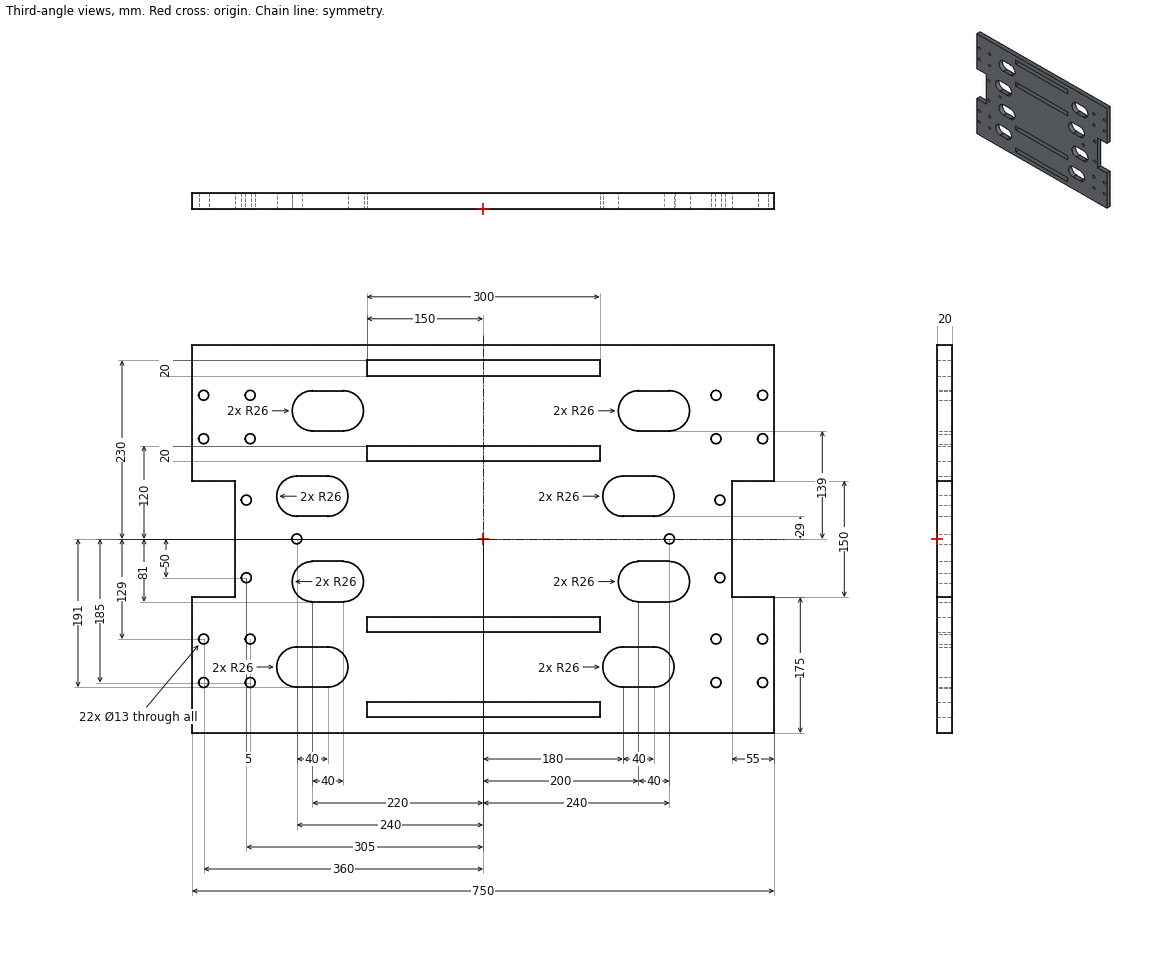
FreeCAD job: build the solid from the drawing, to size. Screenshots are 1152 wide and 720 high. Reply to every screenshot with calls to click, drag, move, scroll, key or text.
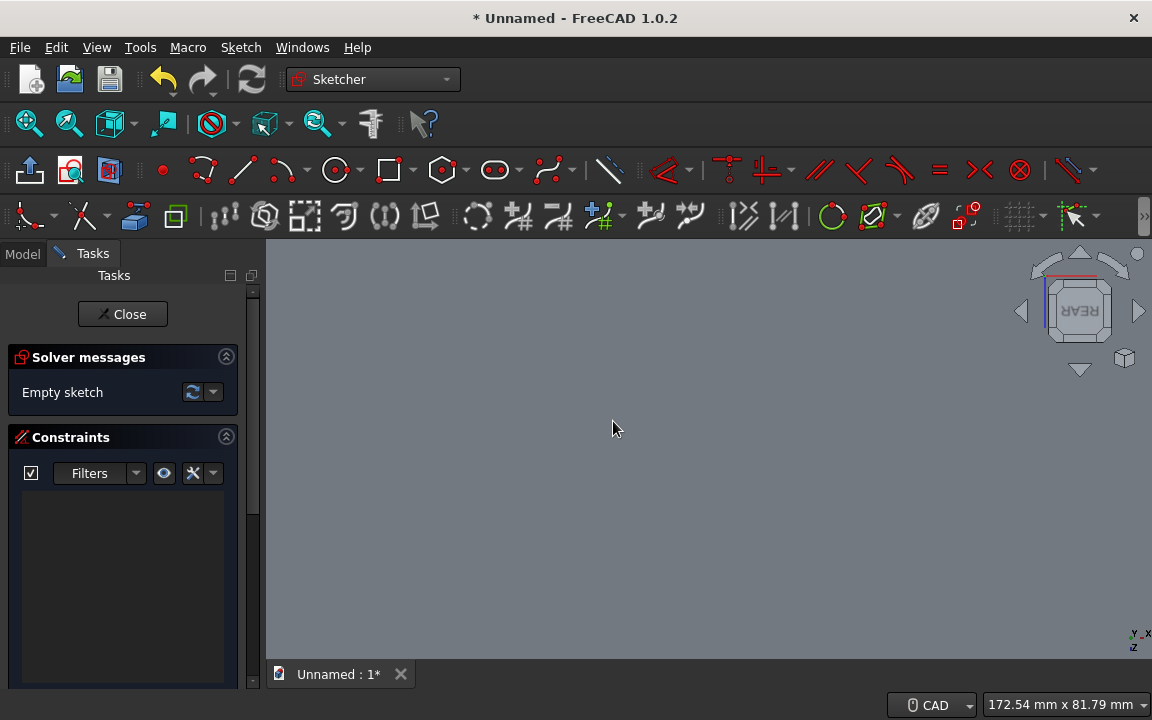
click(496, 170)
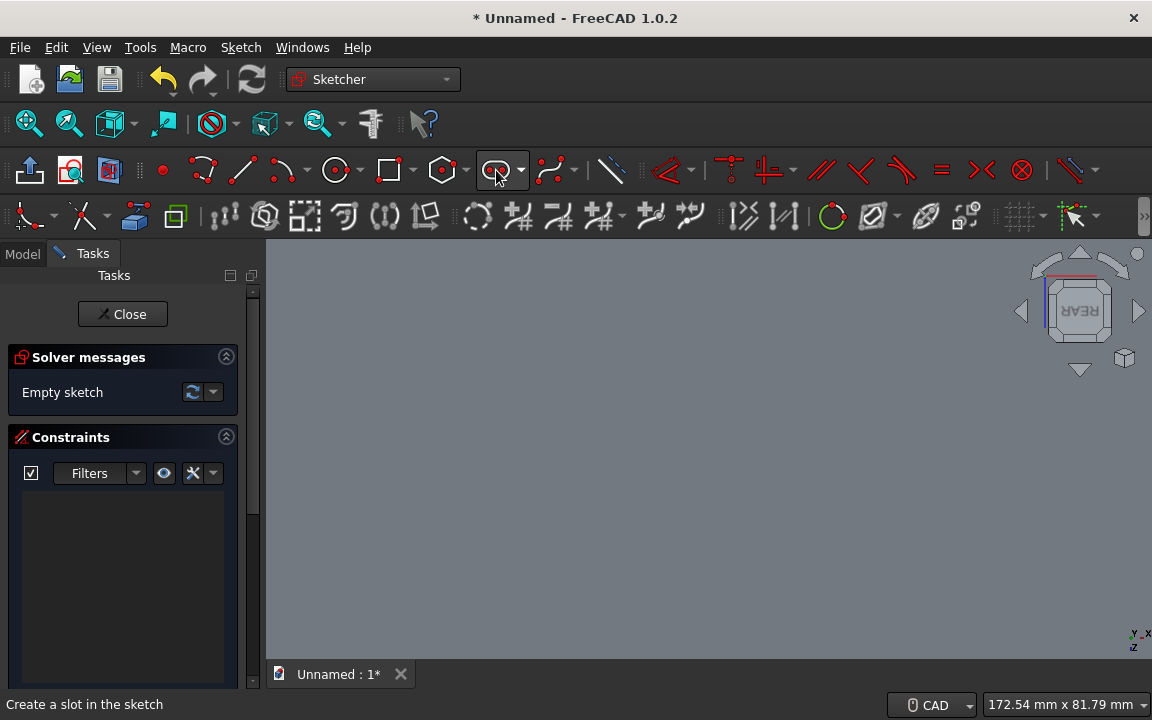
click(538, 443)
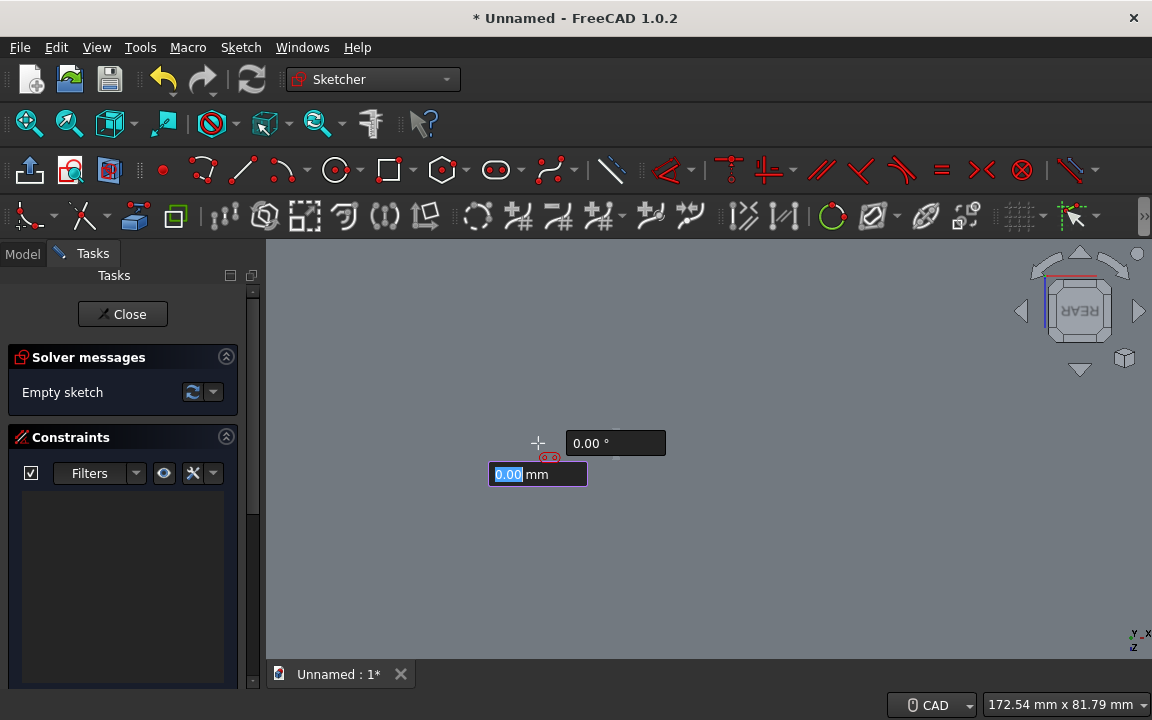
click(743, 443)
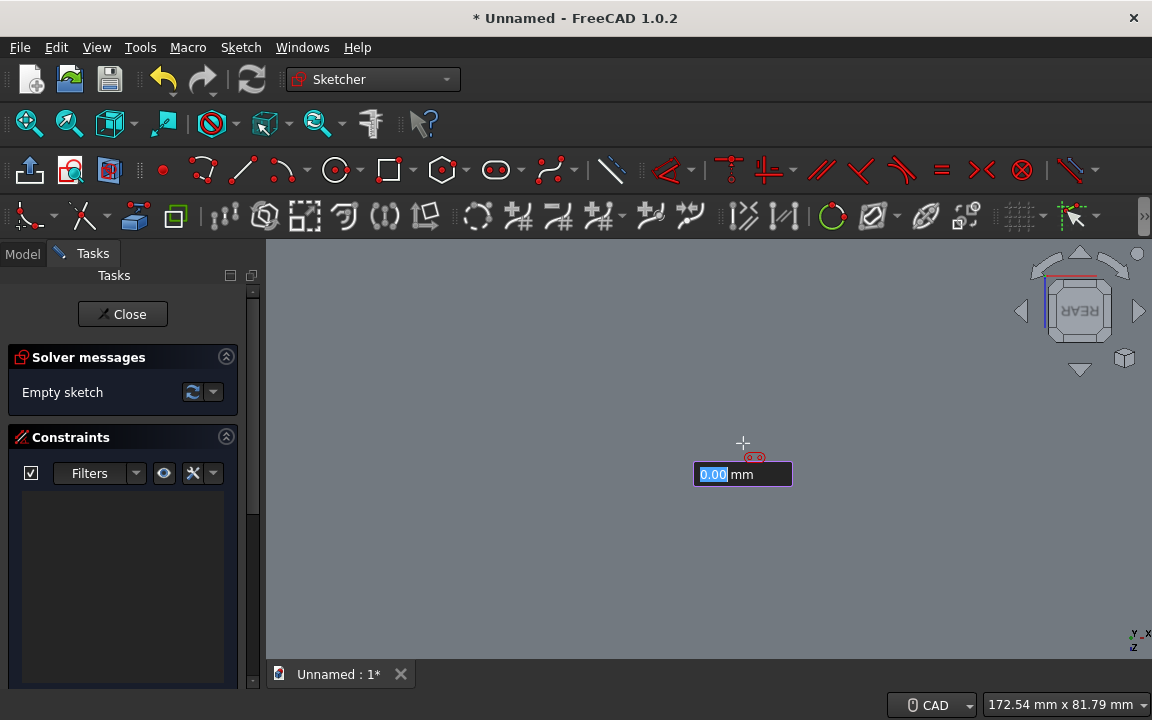
click(640, 309)
key(Escape)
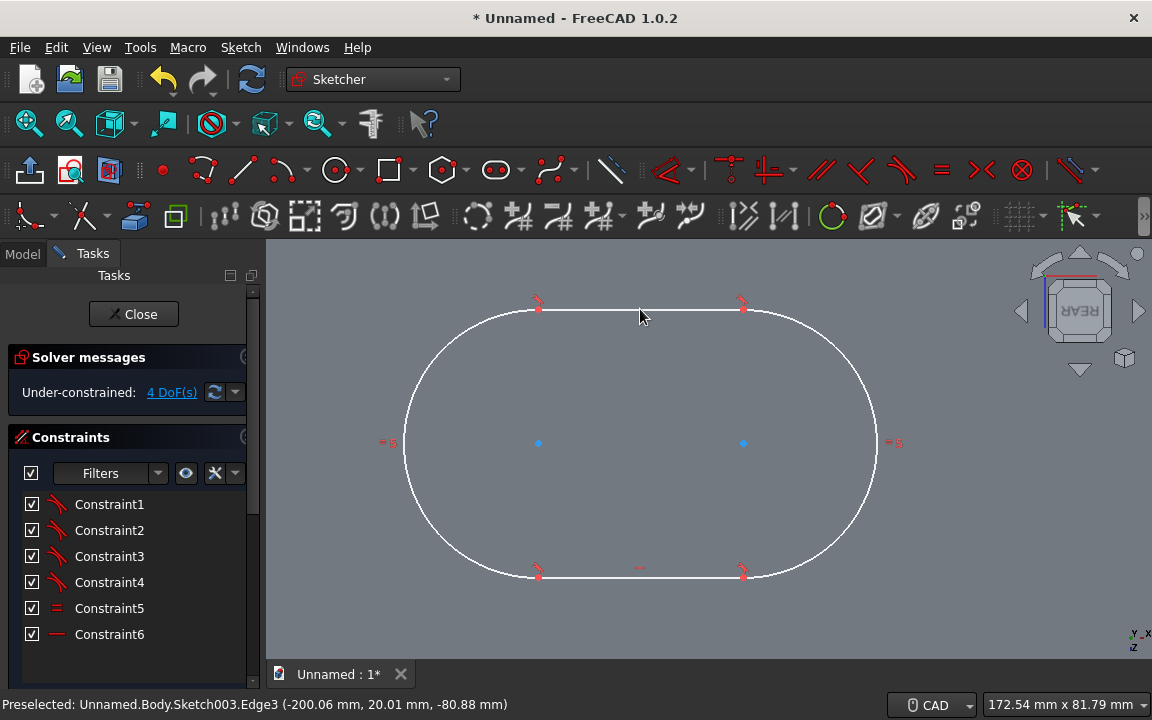
click(666, 170)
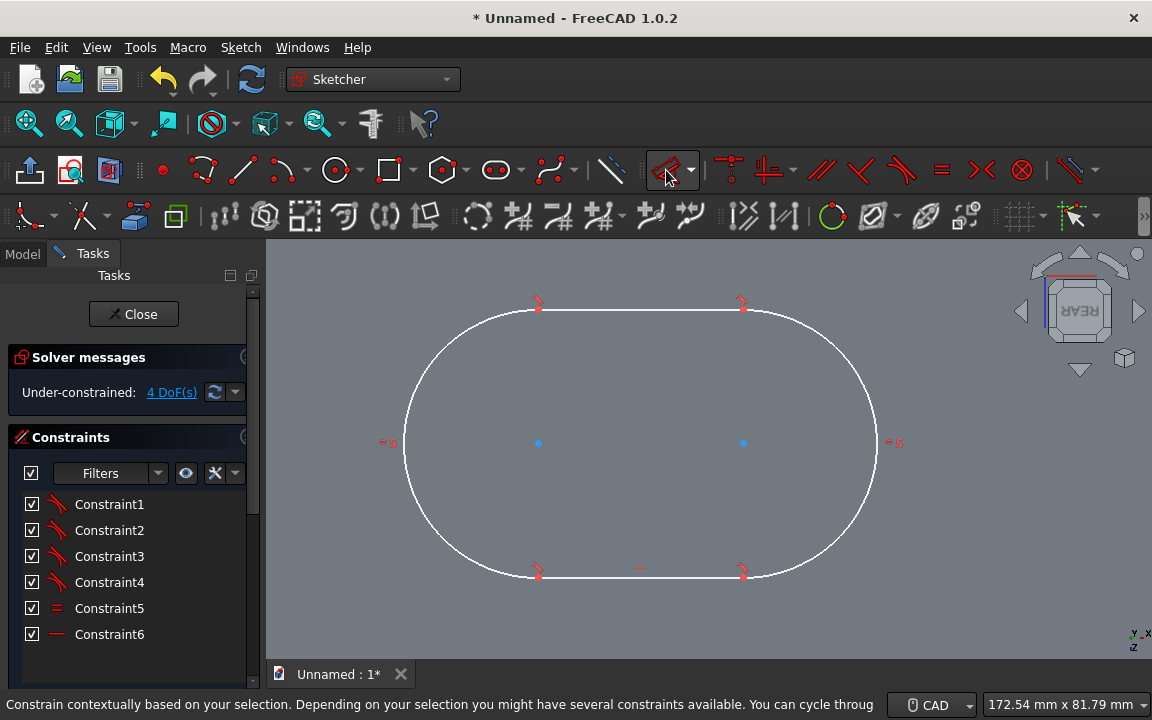
click(430, 365)
click(404, 346)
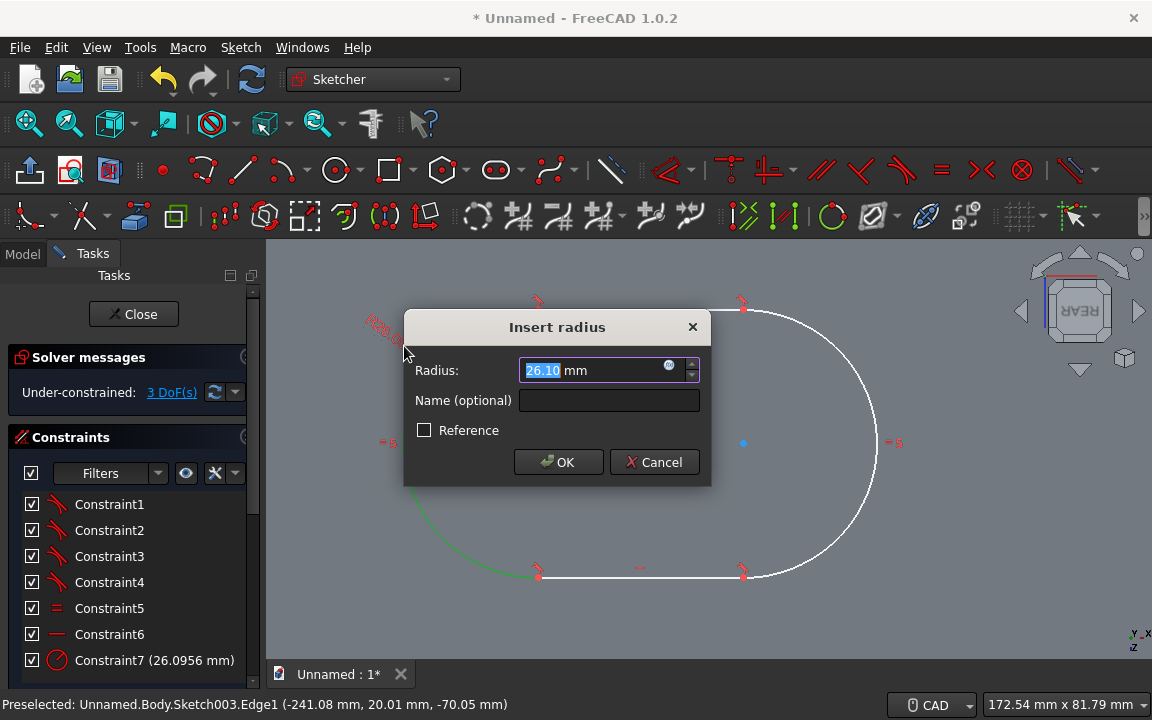
text(26)
key(Return)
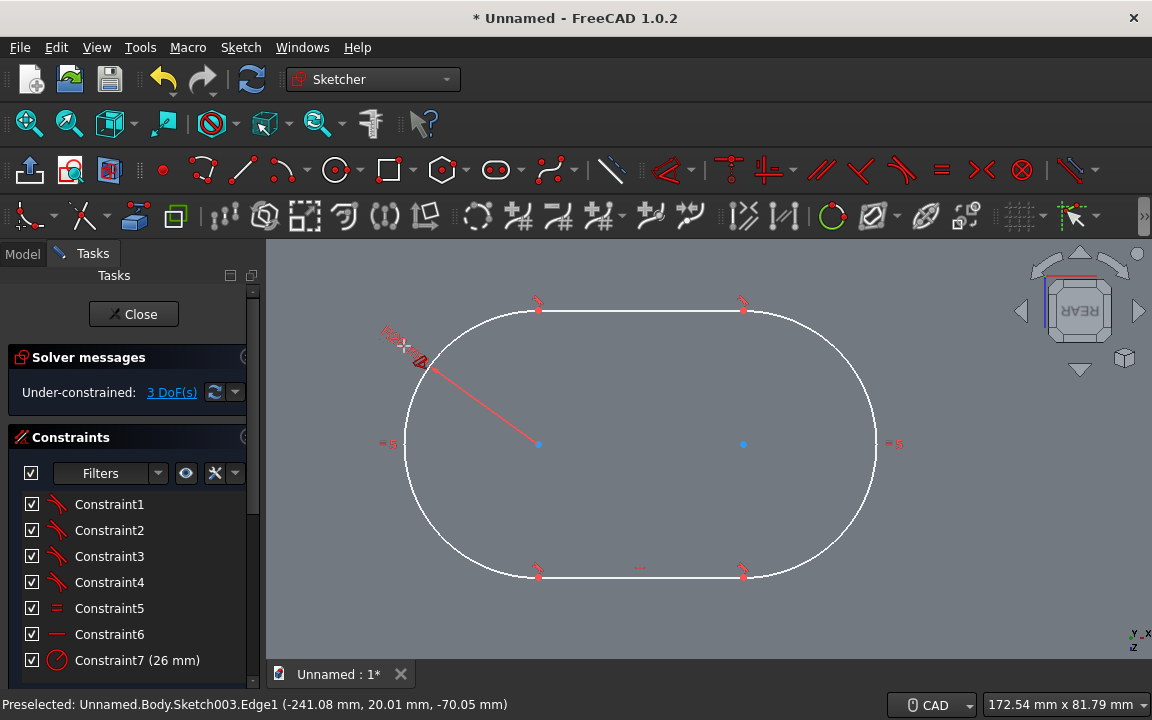
click(600, 311)
click(641, 277)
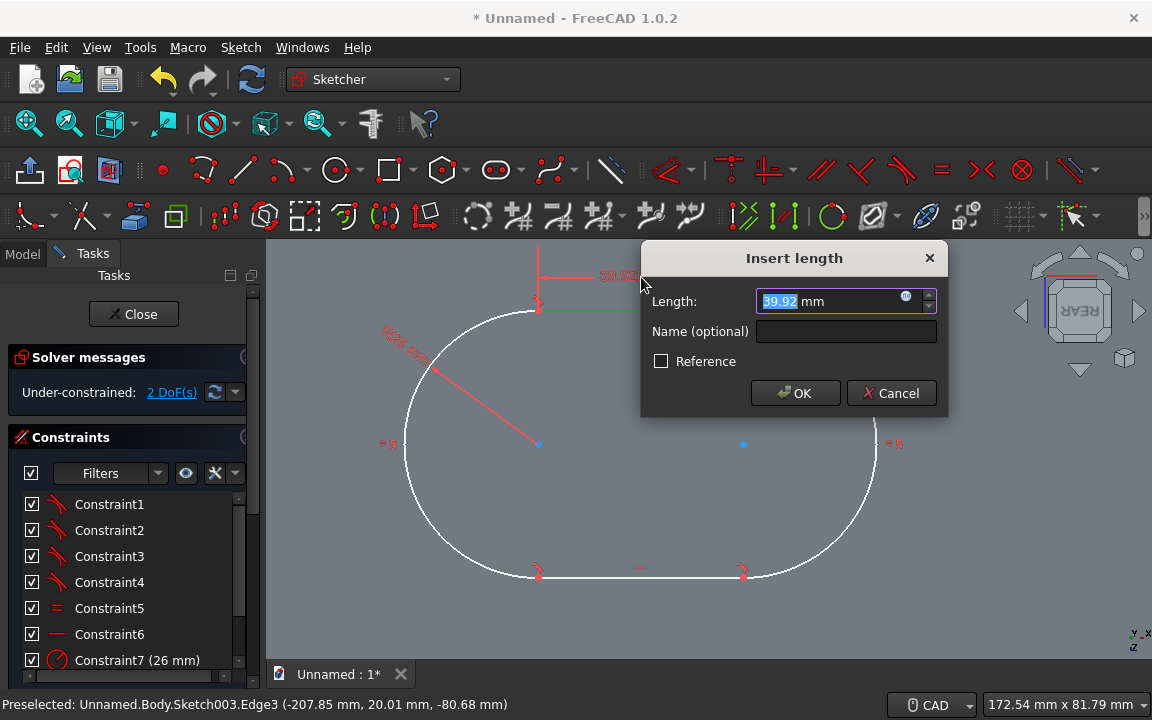
text(40)
key(Return)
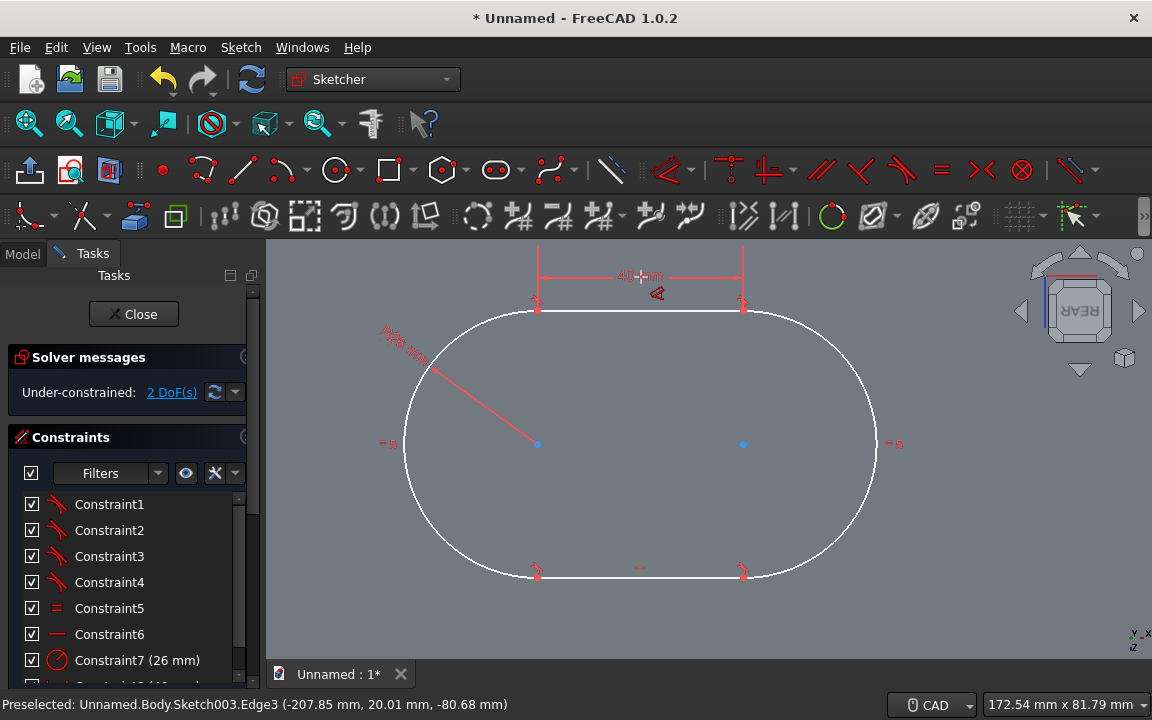
click(538, 311)
click(504, 471)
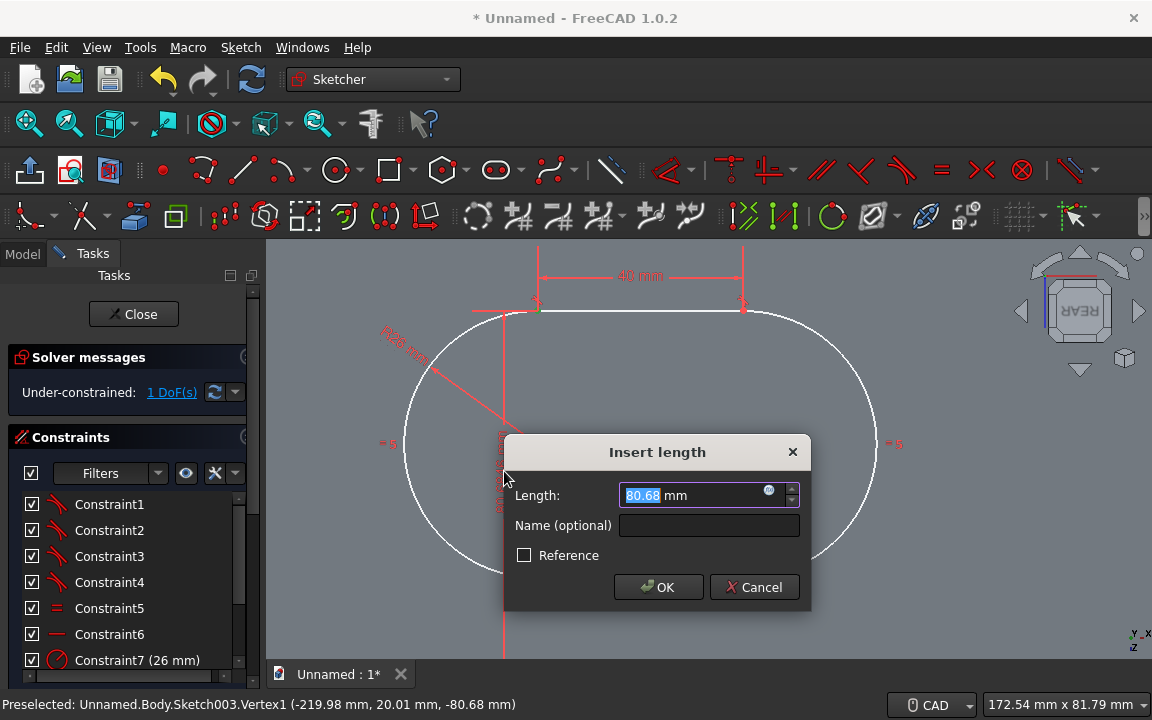
text(81)
key(Return)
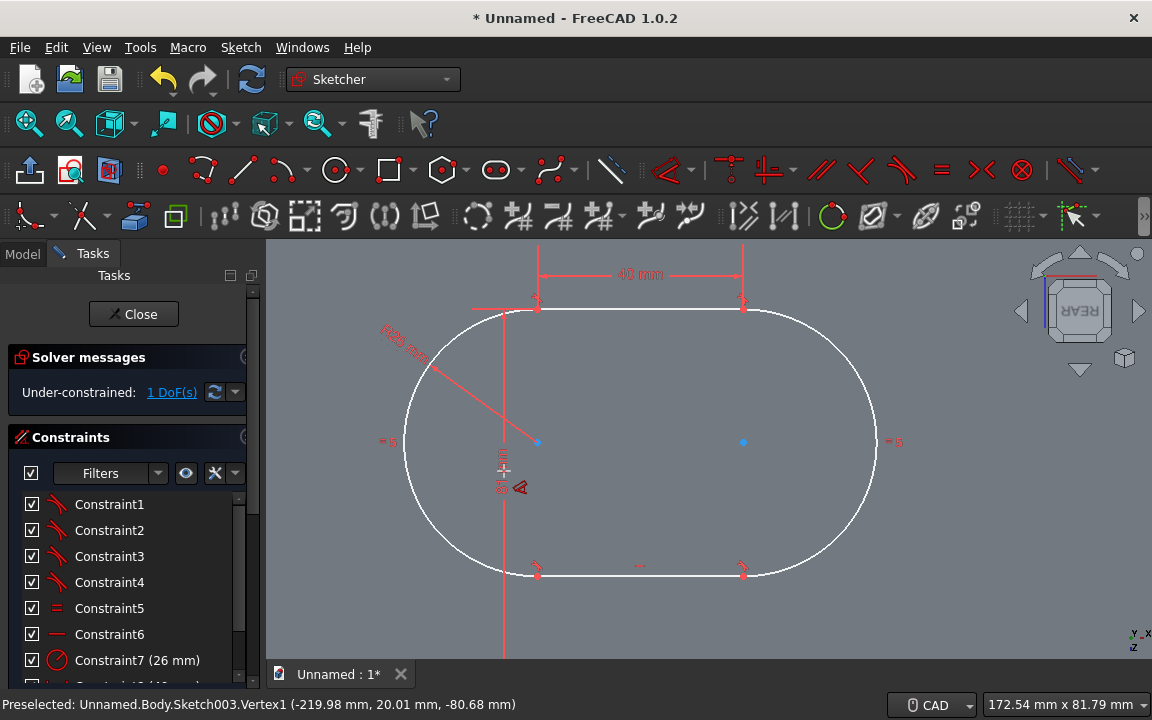
click(538, 309)
click(762, 275)